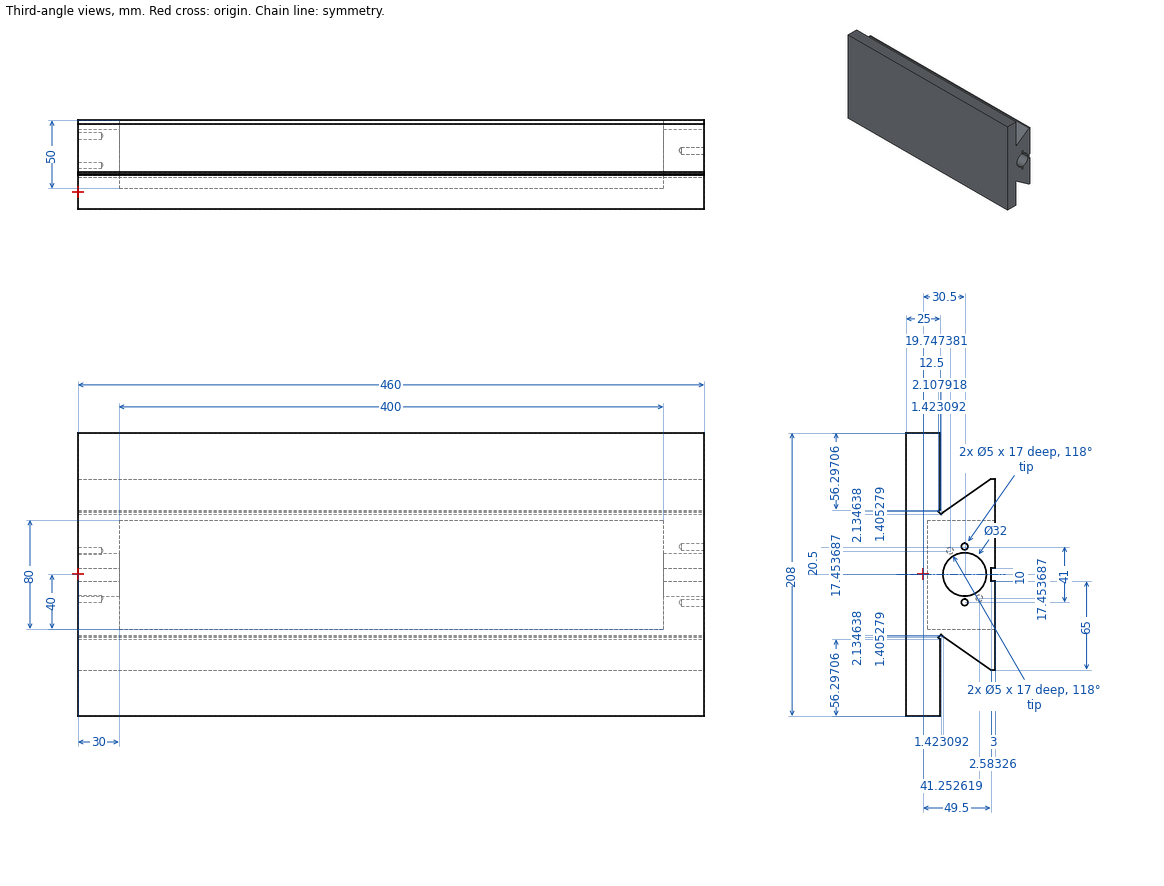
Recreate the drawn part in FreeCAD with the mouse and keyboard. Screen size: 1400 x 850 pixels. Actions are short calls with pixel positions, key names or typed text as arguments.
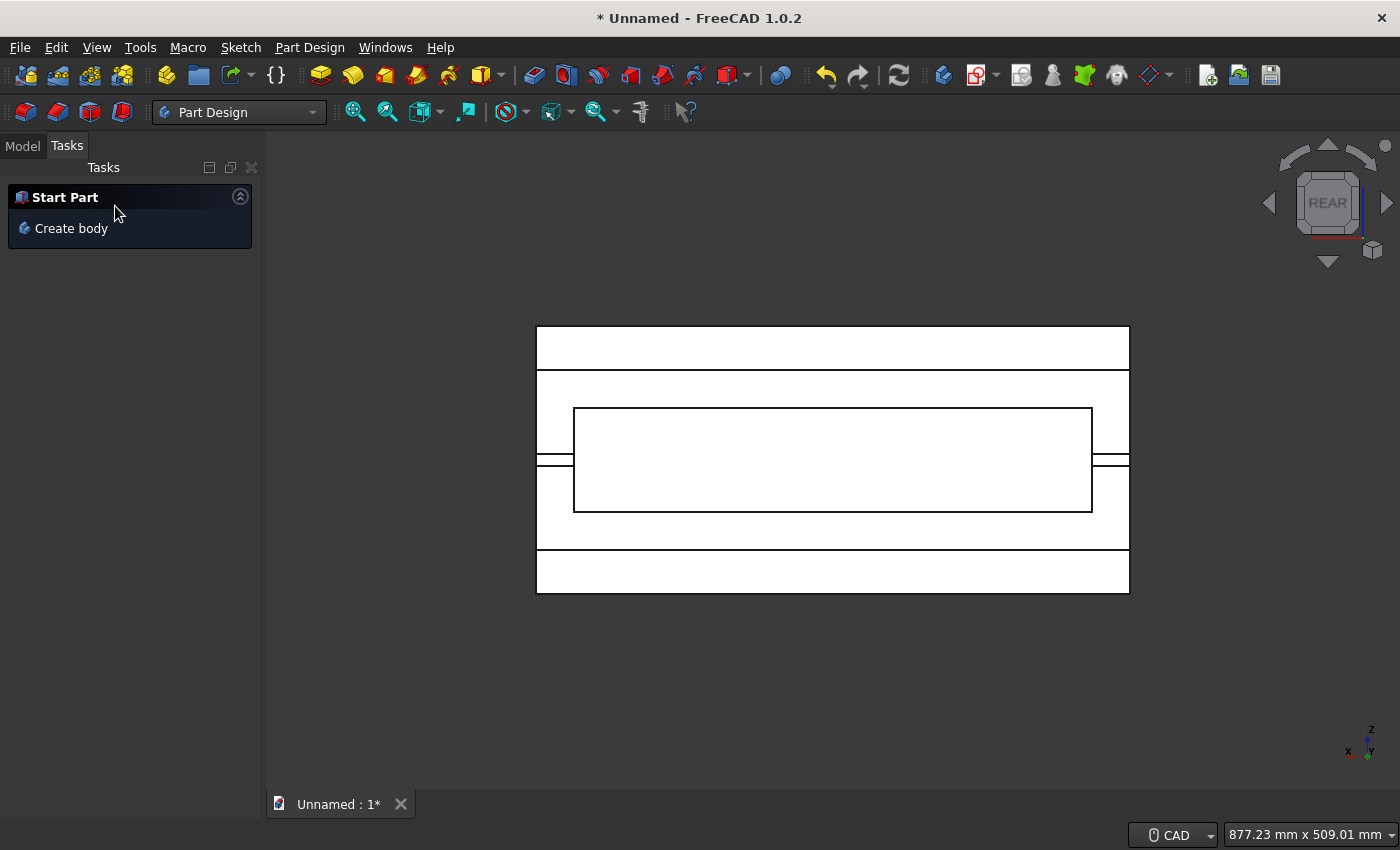
key(0)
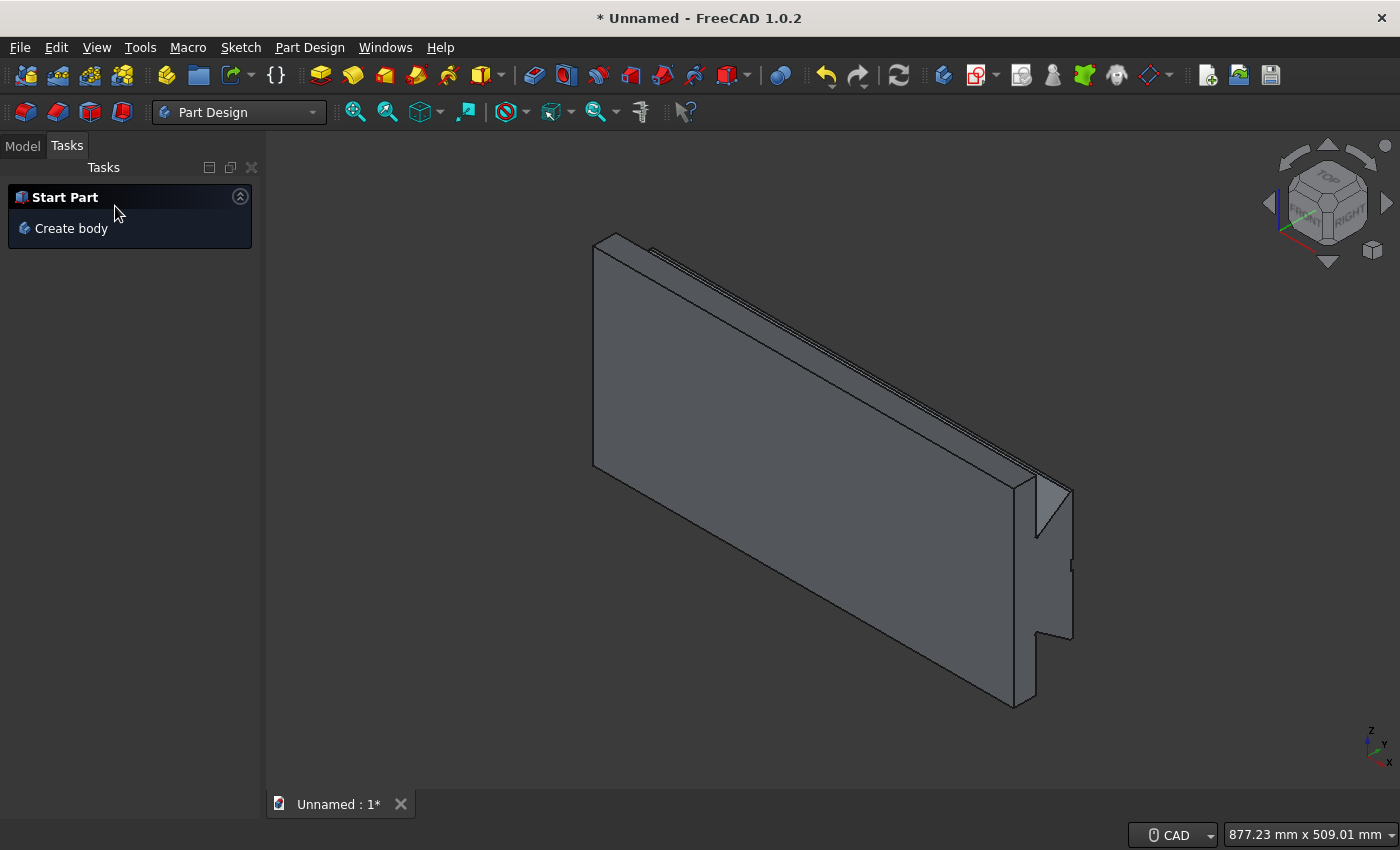
click(1043, 580)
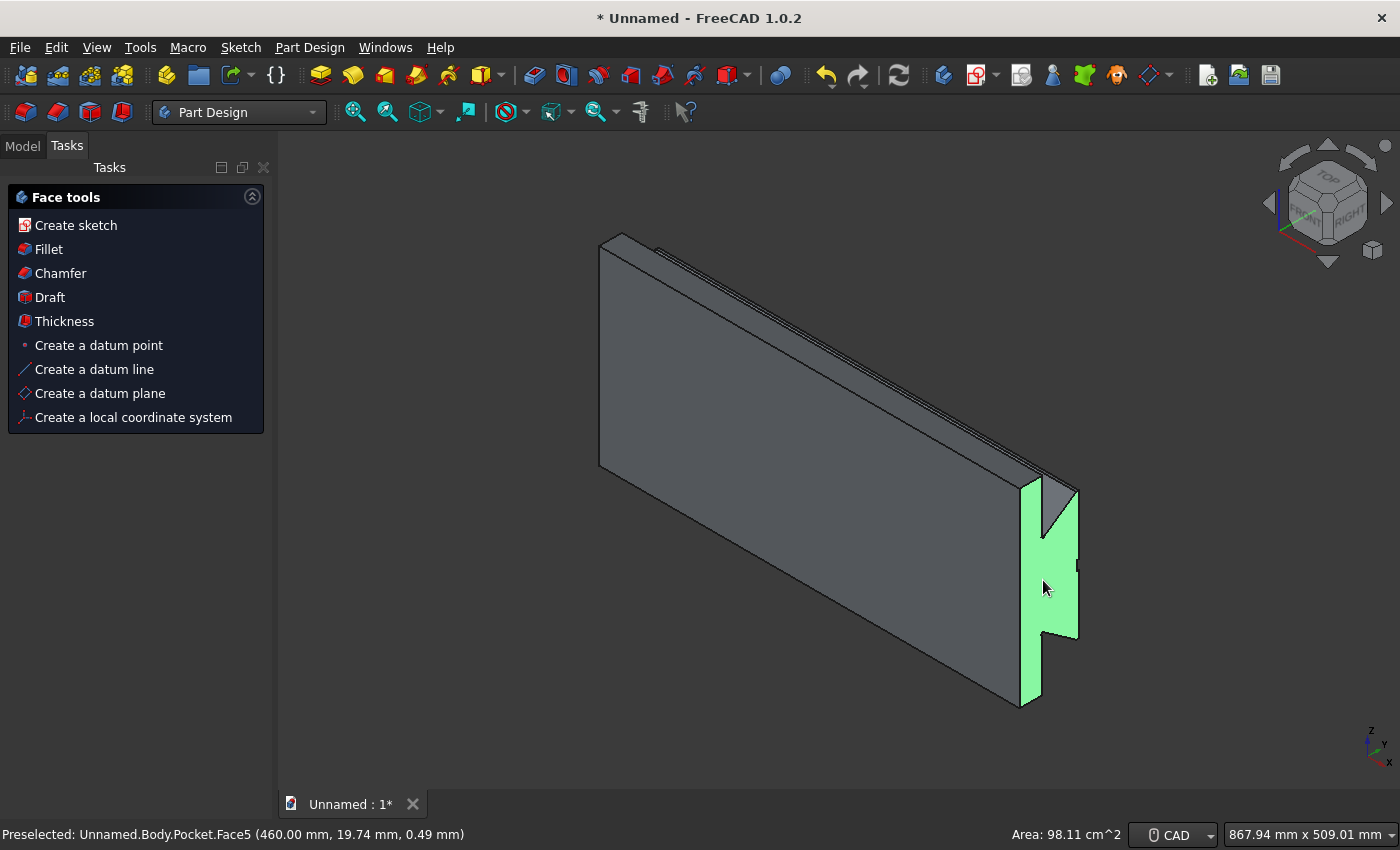
click(976, 76)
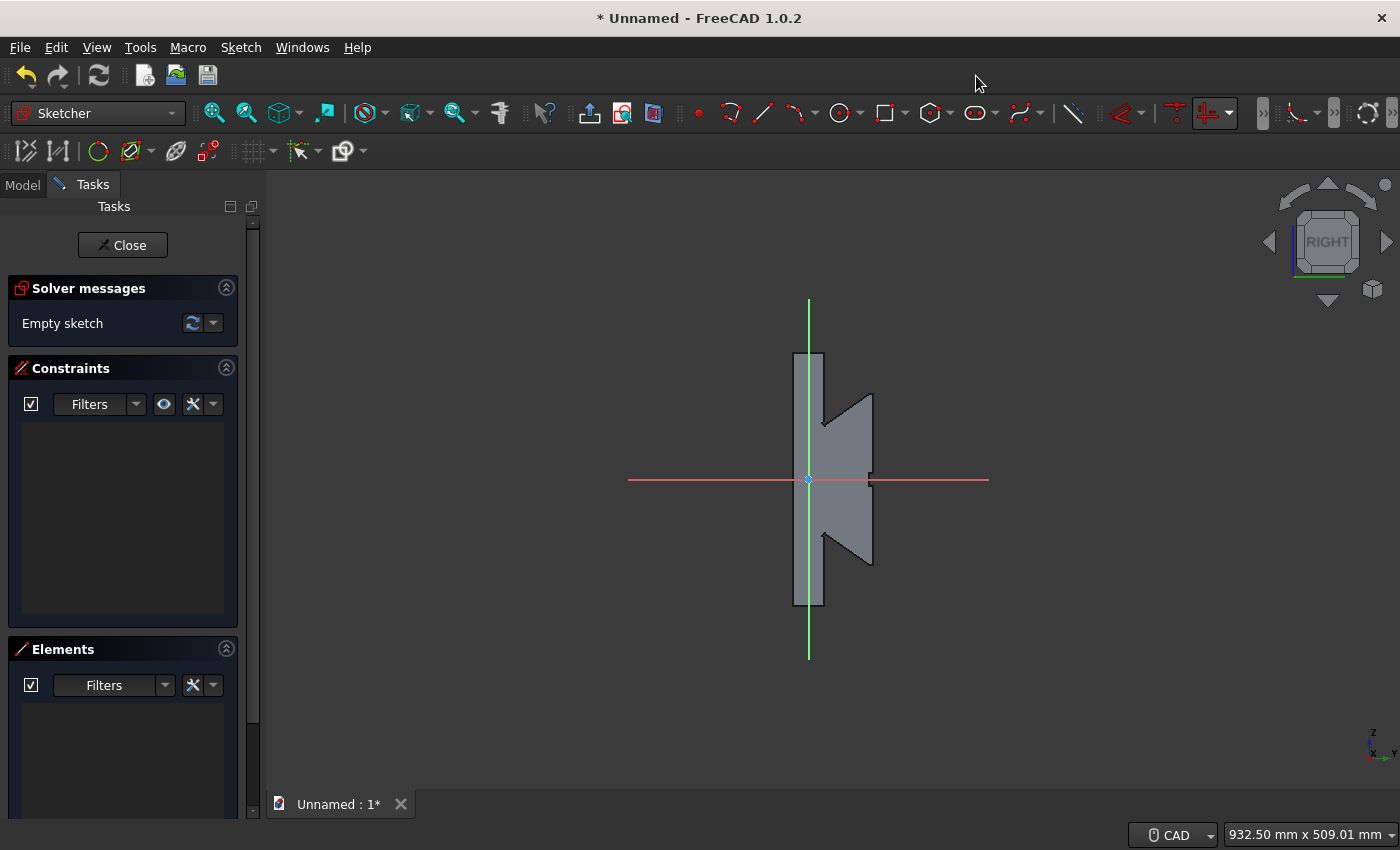
scroll(844, 480, up, 12)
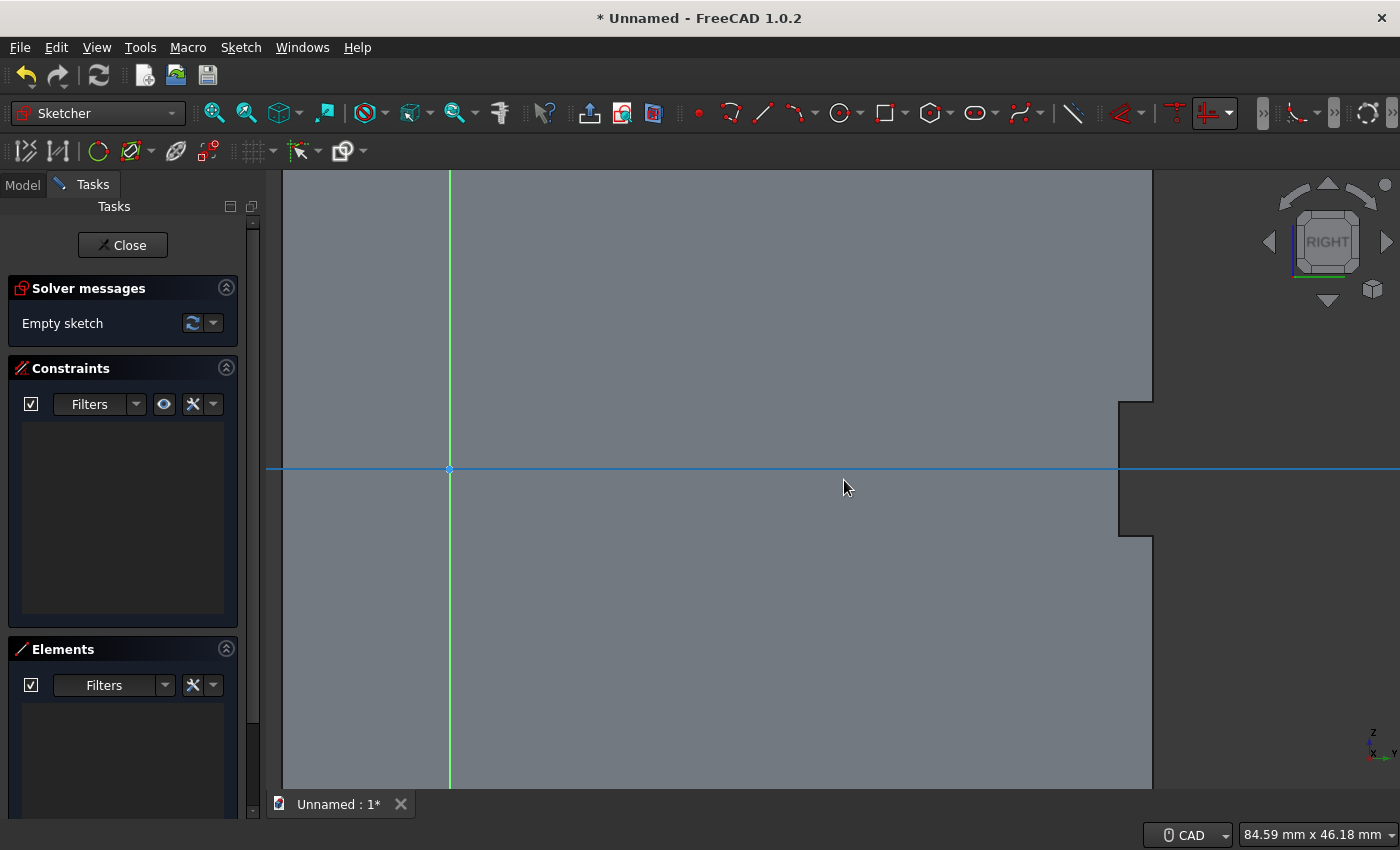
click(840, 114)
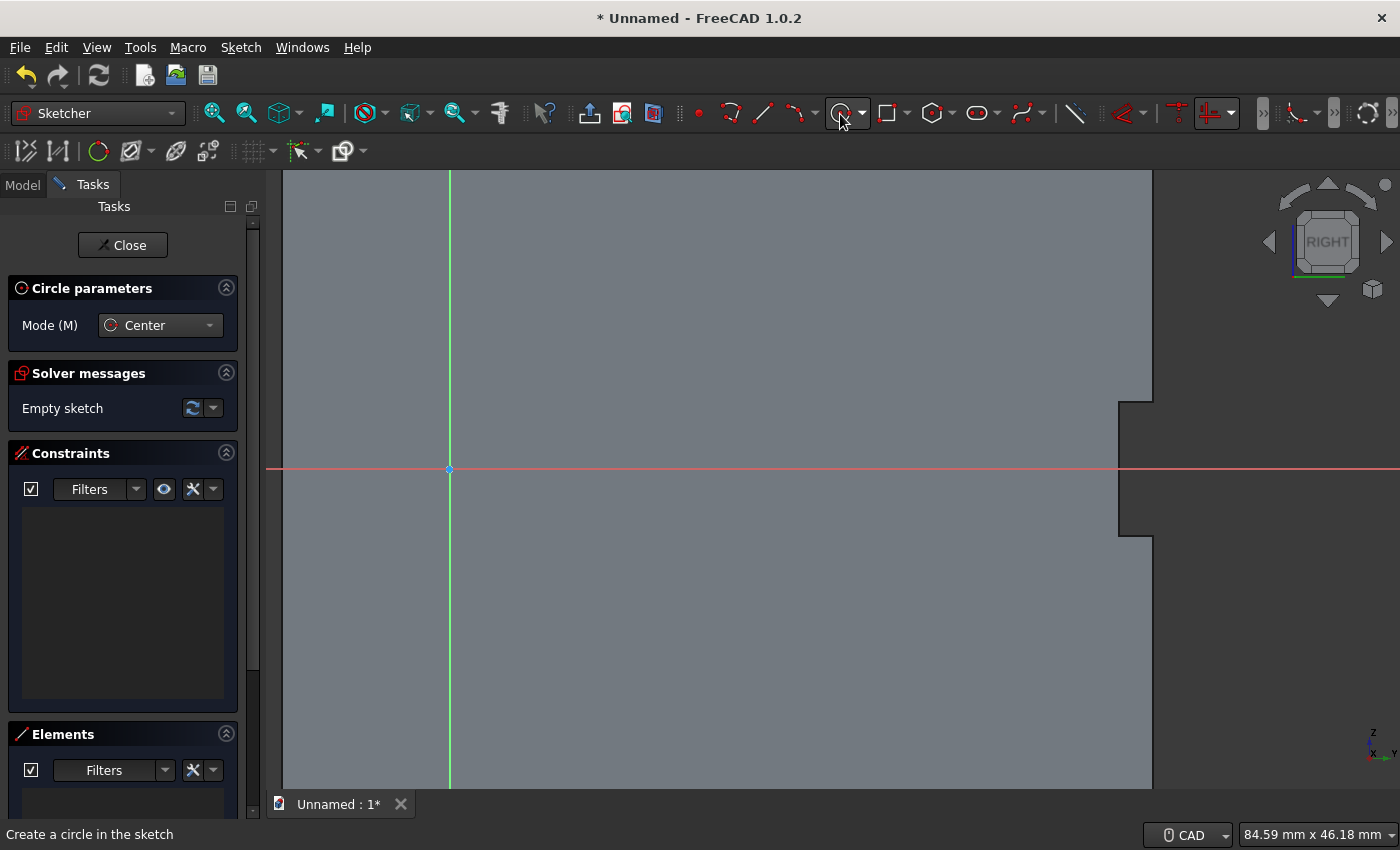
click(858, 469)
move(1010, 318)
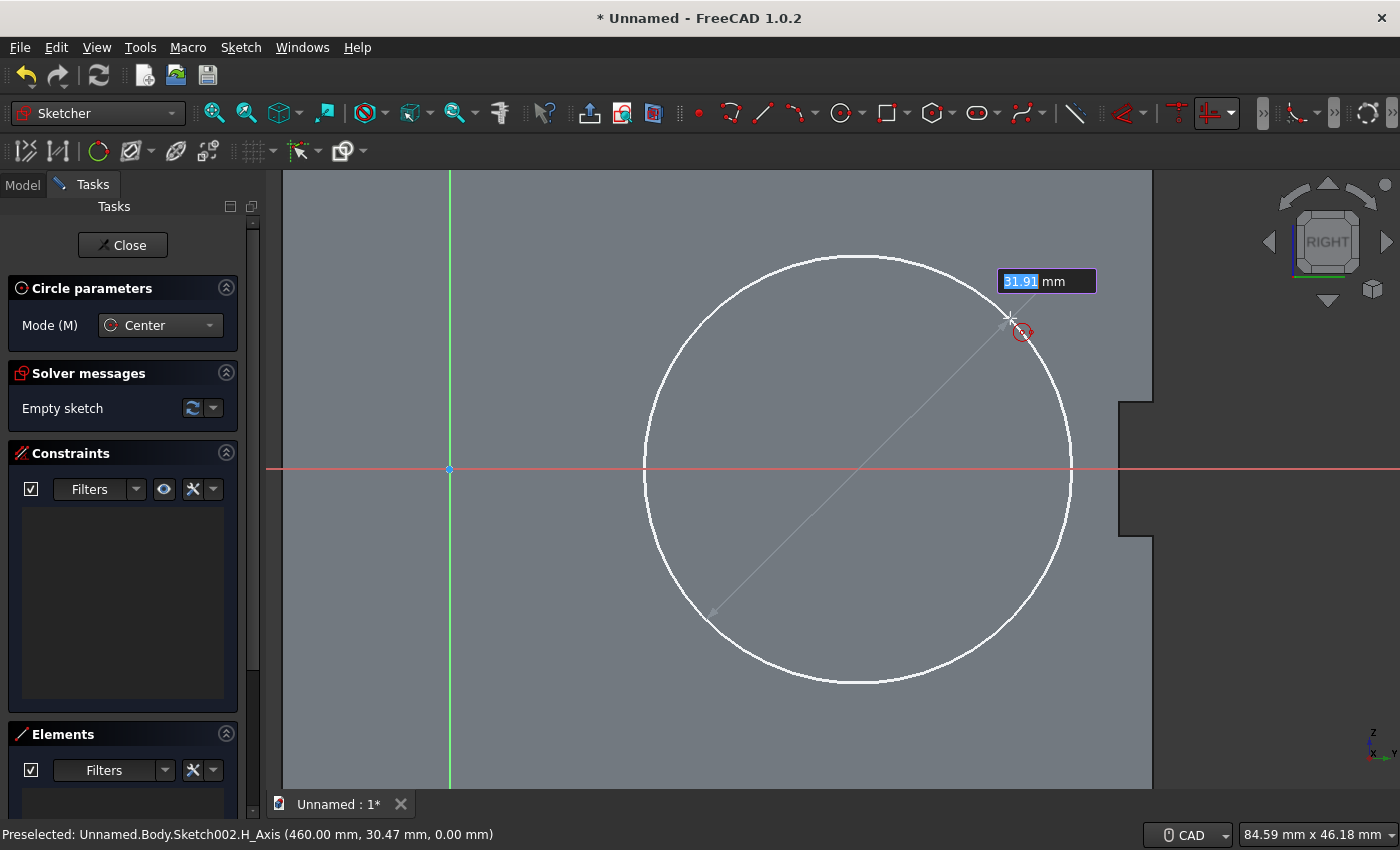
text(32)
key(Return)
key(Escape)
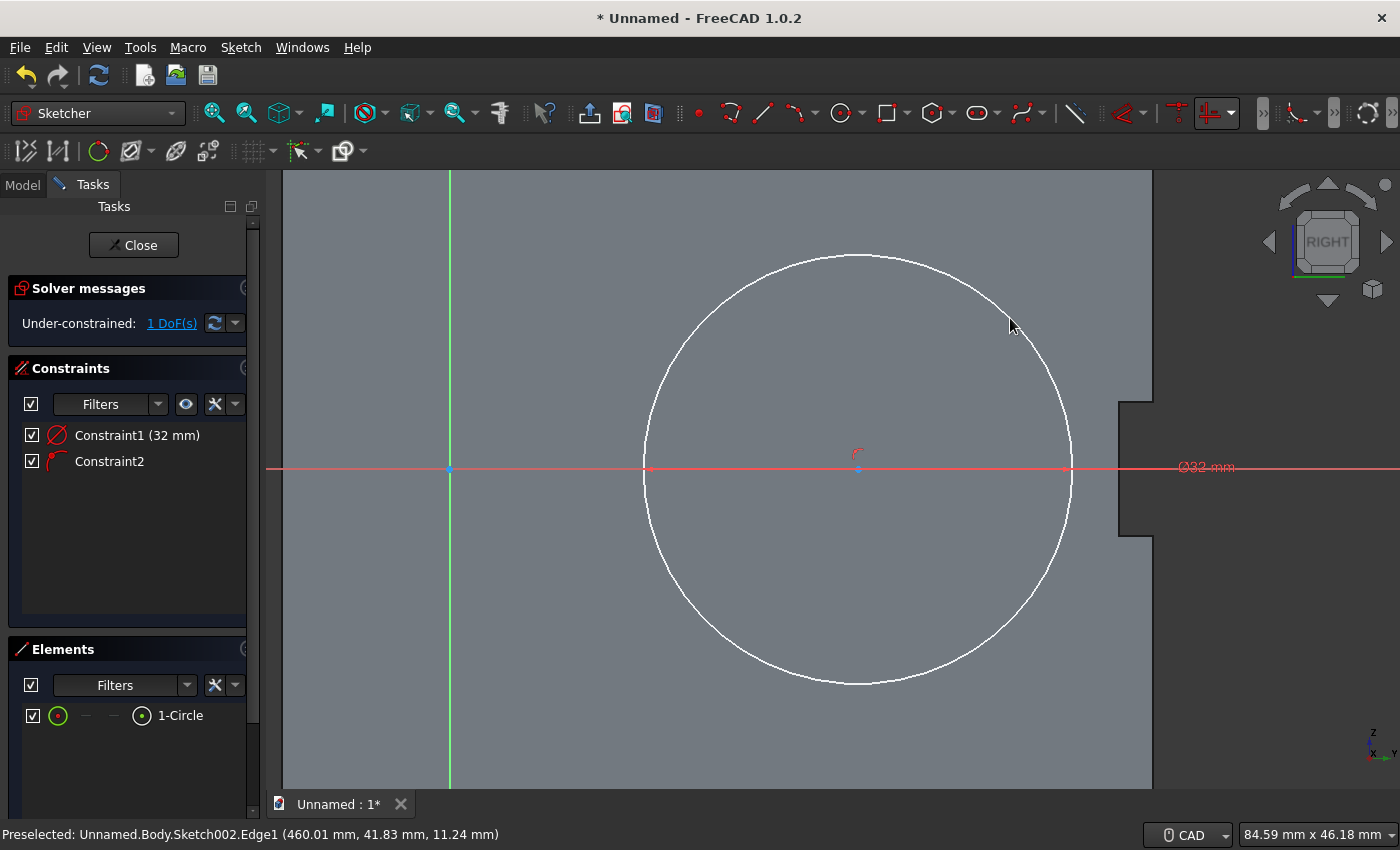
click(1122, 114)